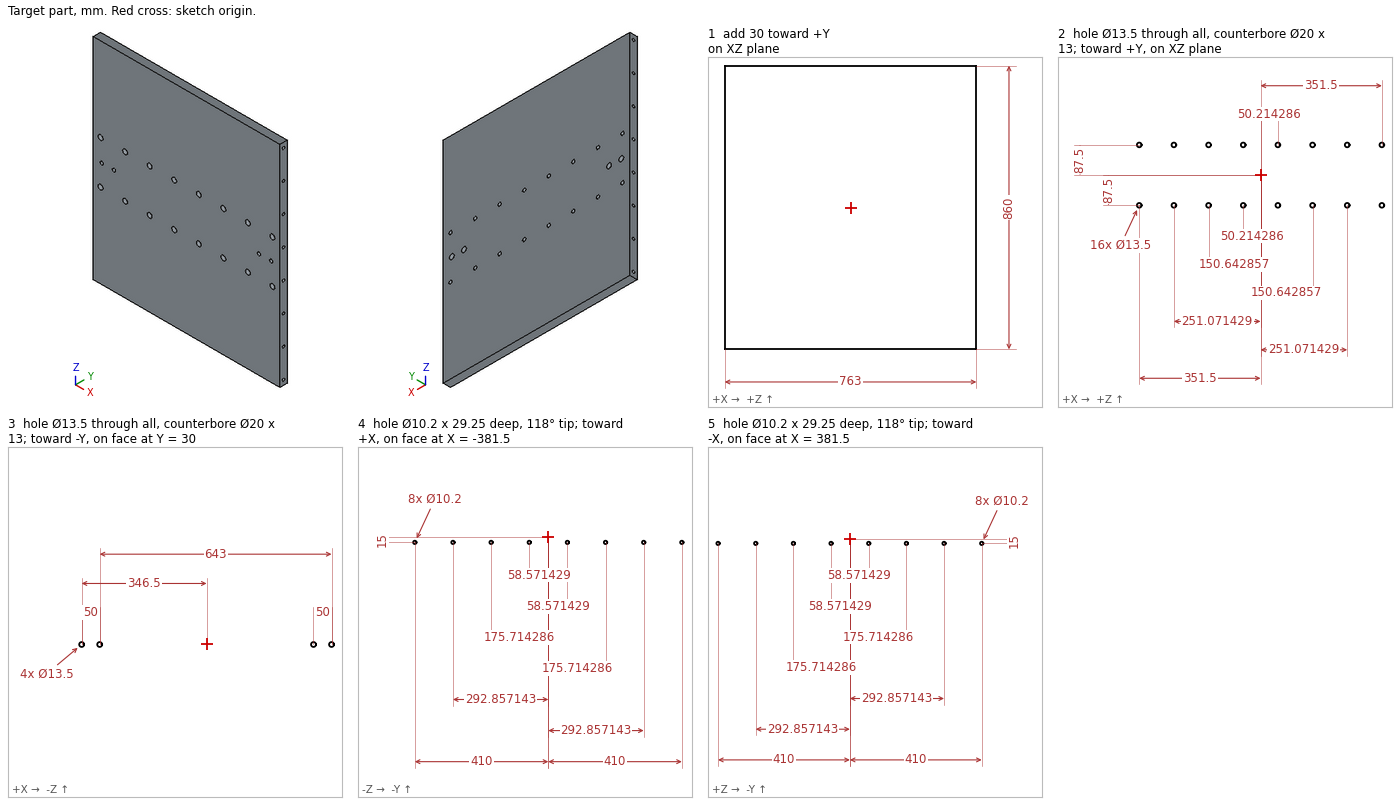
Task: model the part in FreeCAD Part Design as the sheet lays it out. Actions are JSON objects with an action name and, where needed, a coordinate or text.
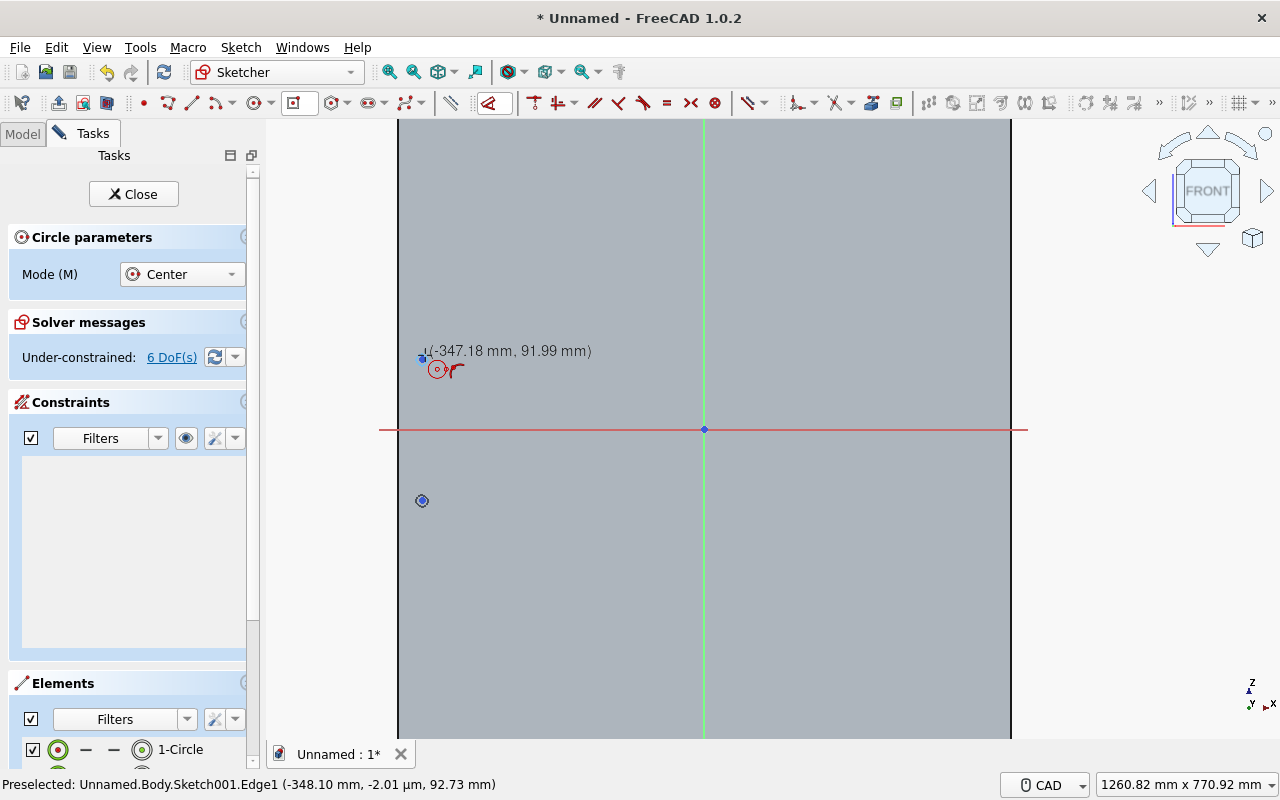
{"action": "scroll", "coordinate": [502, 500], "scroll_direction": "up", "scroll_amount": 8}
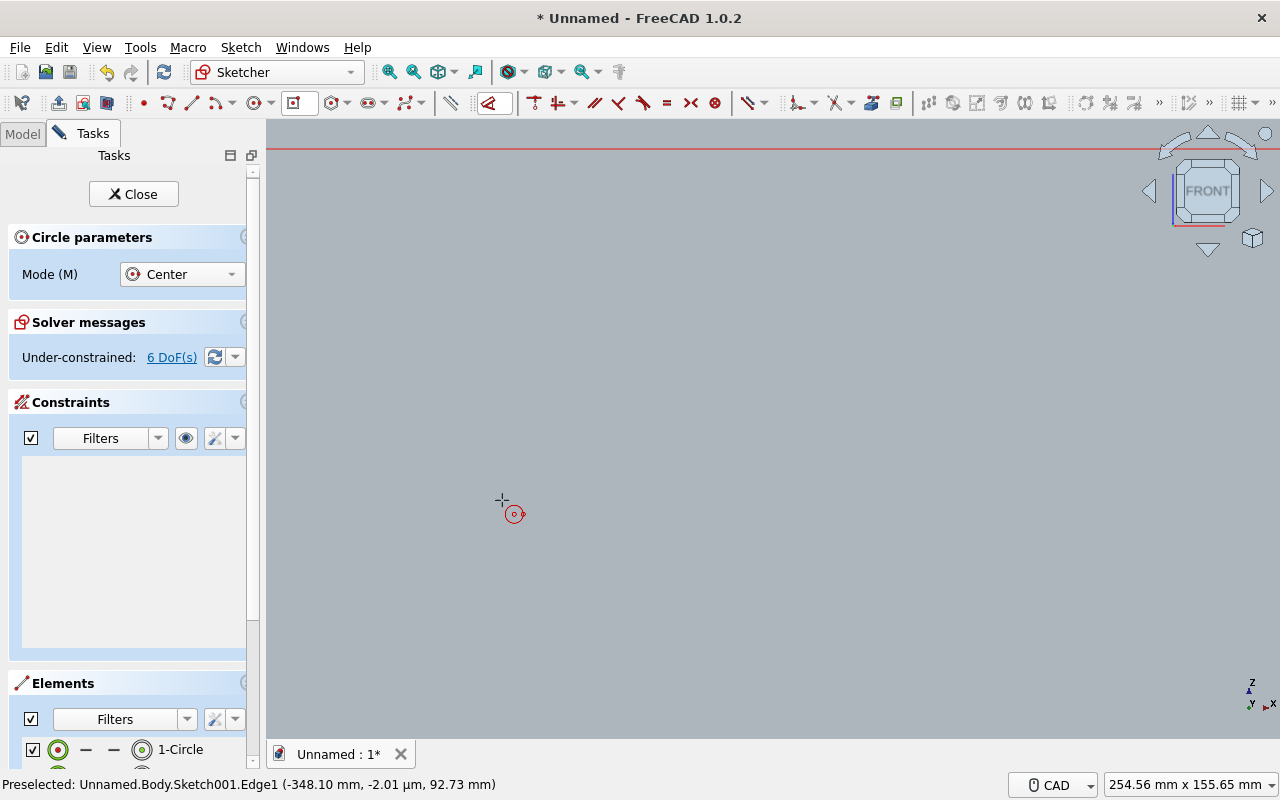
{"action": "scroll", "coordinate": [502, 500], "scroll_direction": "down", "scroll_amount": 8}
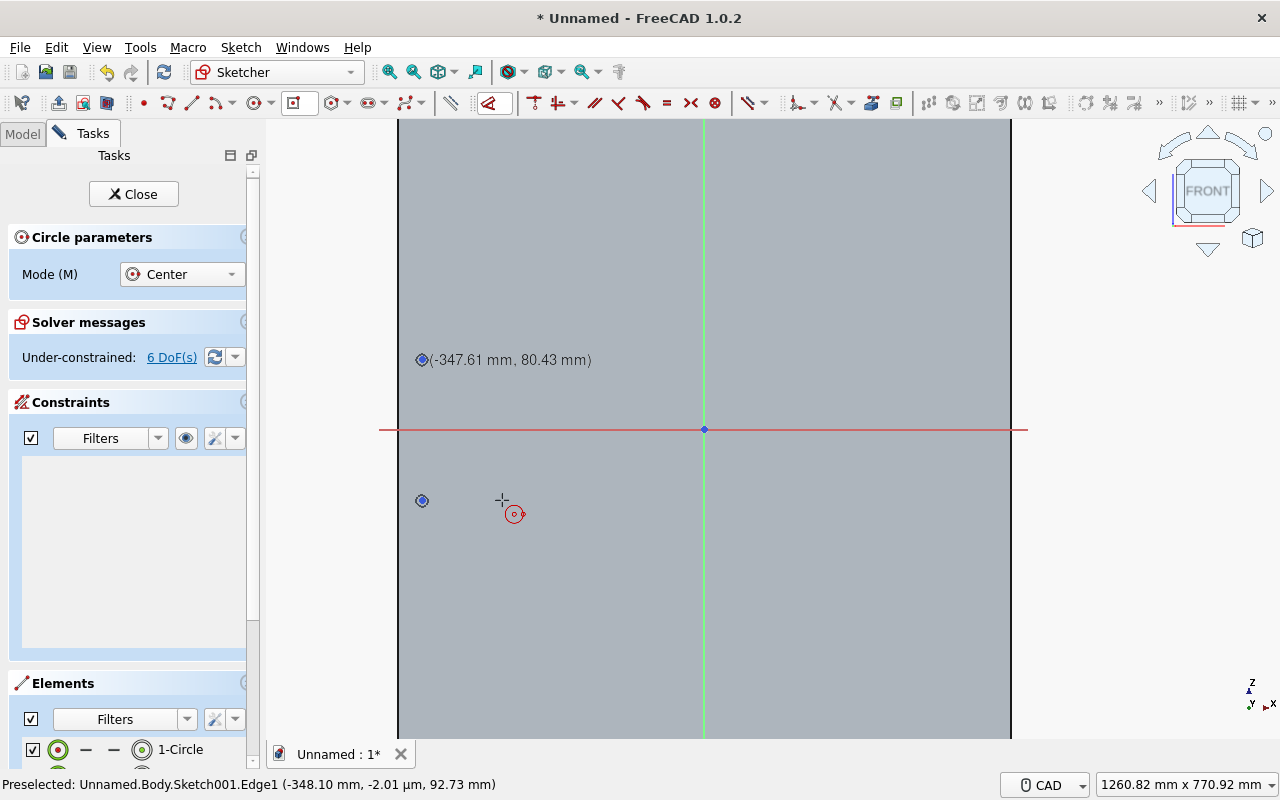
{"action": "left_click", "coordinate": [502, 500]}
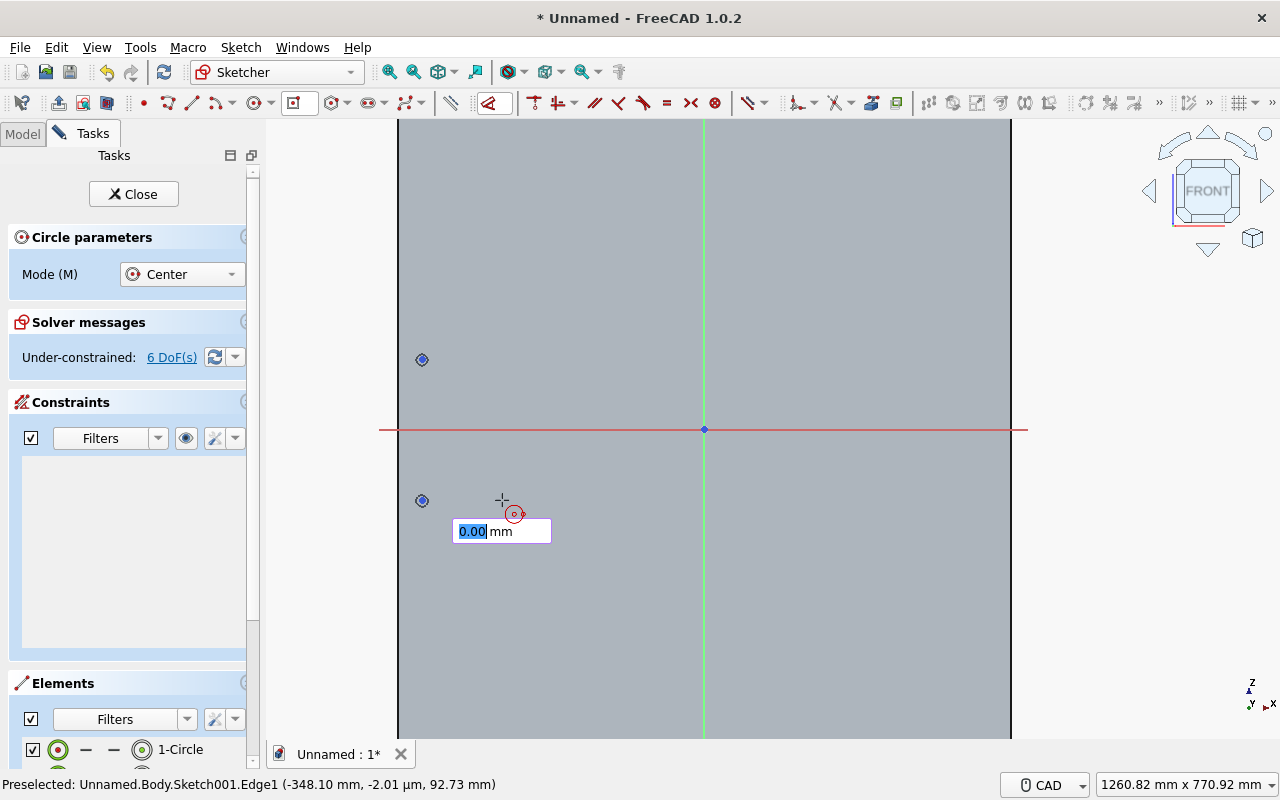
{"action": "scroll", "coordinate": [506, 496], "scroll_direction": "up", "scroll_amount": 6}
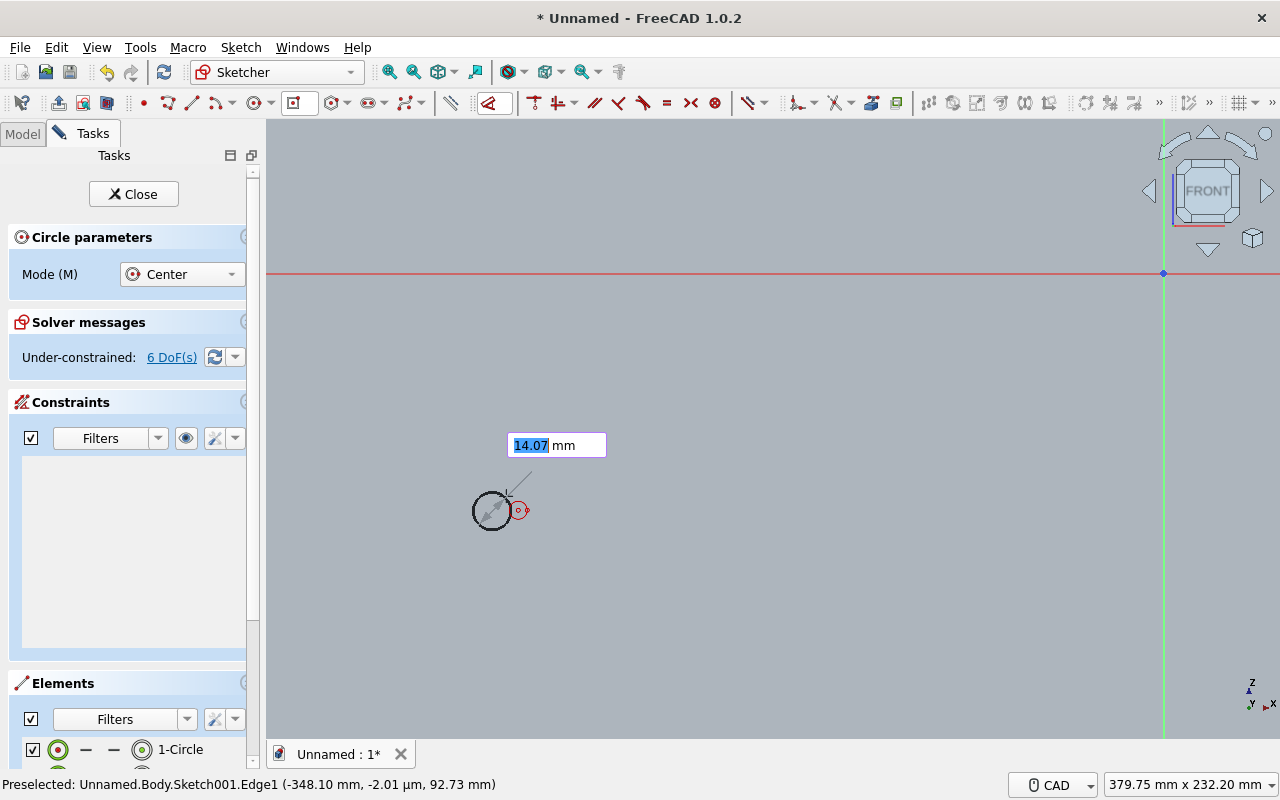
{"action": "left_click", "coordinate": [506, 495]}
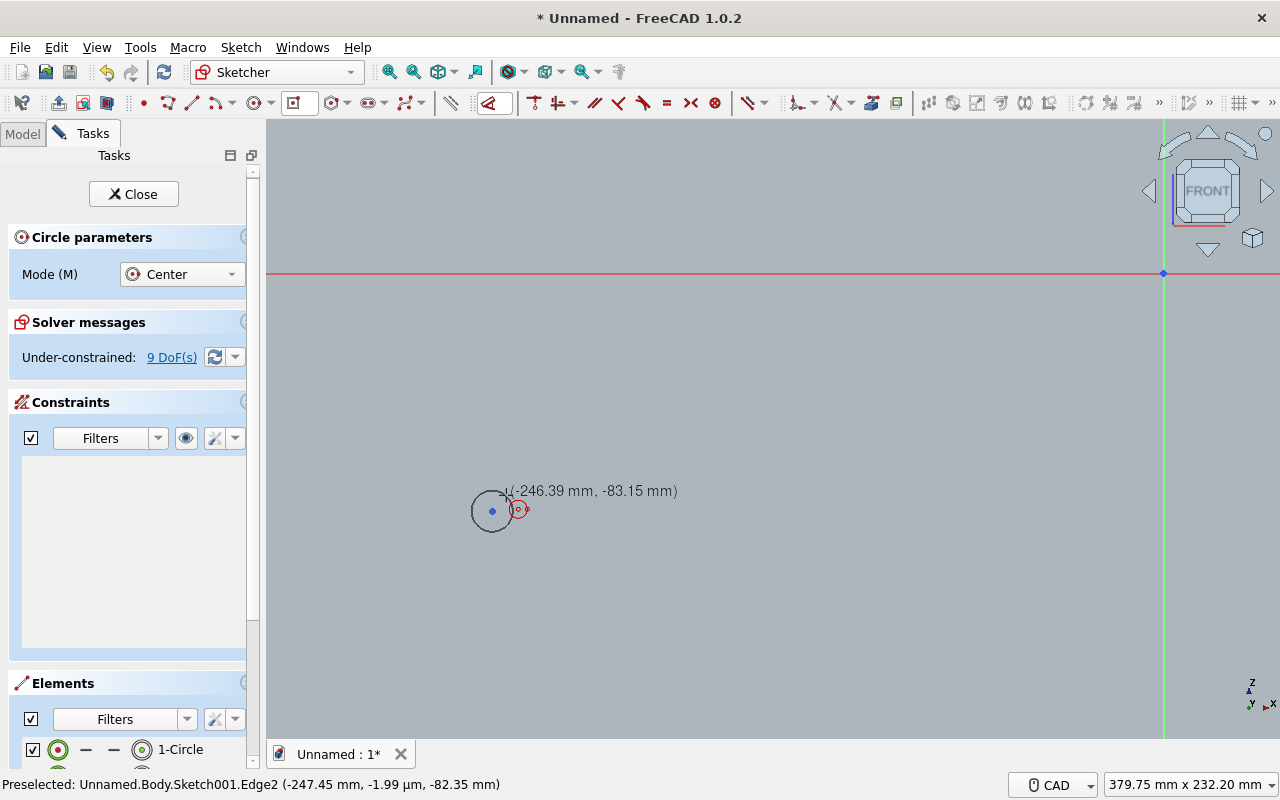
{"action": "scroll", "coordinate": [506, 496], "scroll_direction": "down", "scroll_amount": 6}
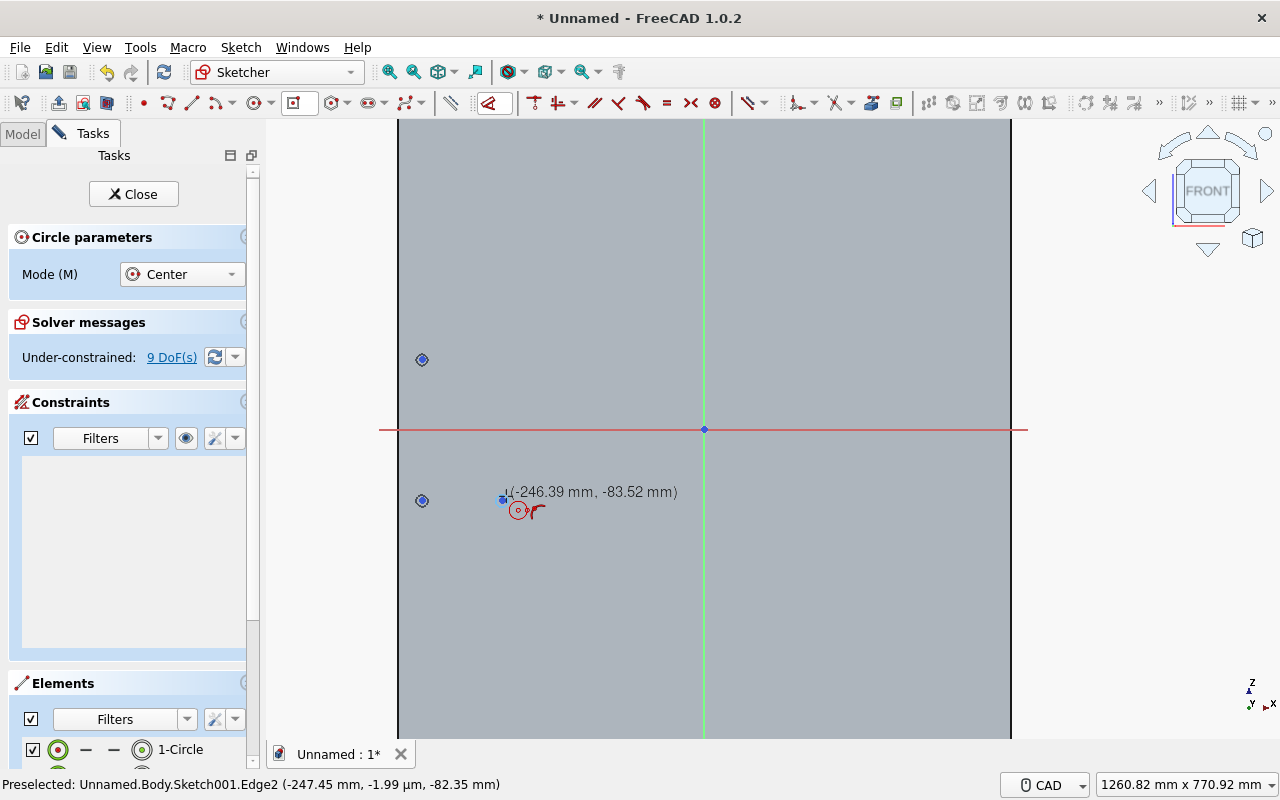
{"action": "scroll", "coordinate": [502, 359], "scroll_direction": "up", "scroll_amount": 8}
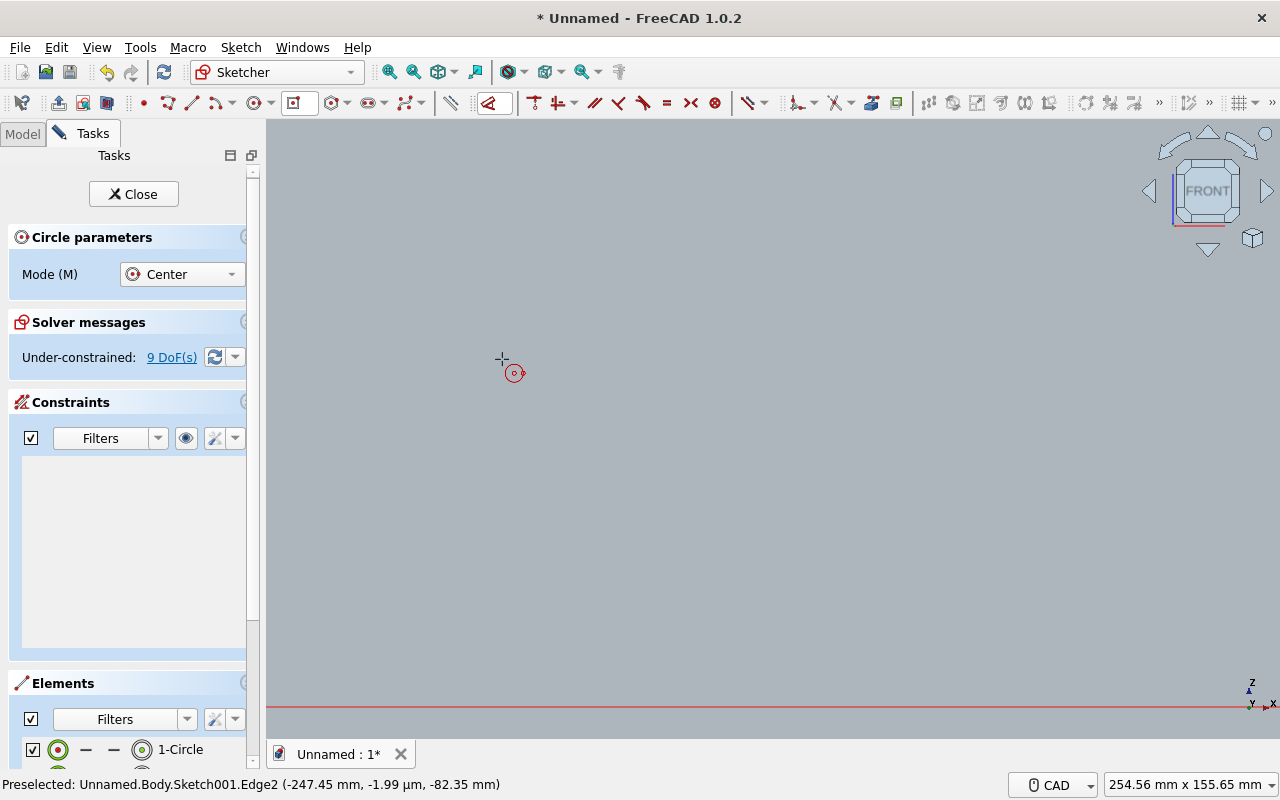
{"action": "scroll", "coordinate": [502, 359], "scroll_direction": "down", "scroll_amount": 8}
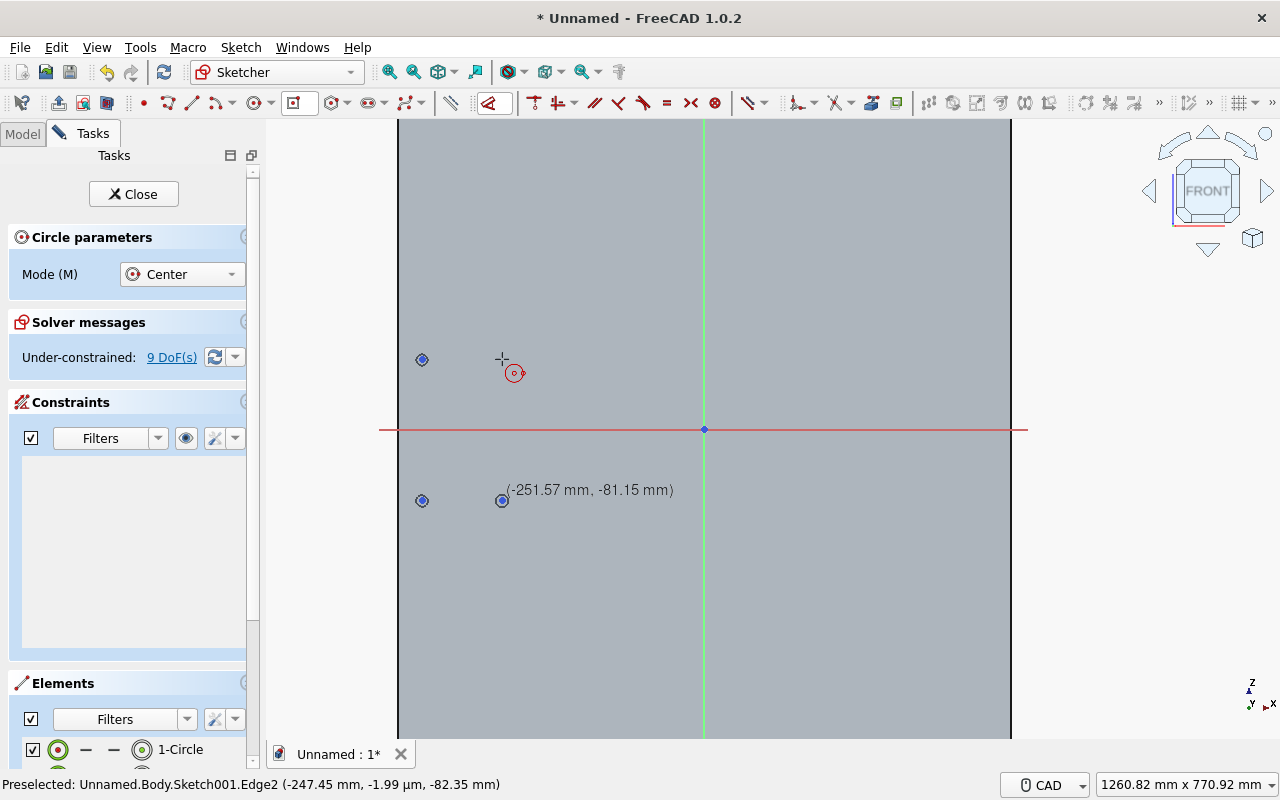
{"action": "left_click", "coordinate": [502, 359]}